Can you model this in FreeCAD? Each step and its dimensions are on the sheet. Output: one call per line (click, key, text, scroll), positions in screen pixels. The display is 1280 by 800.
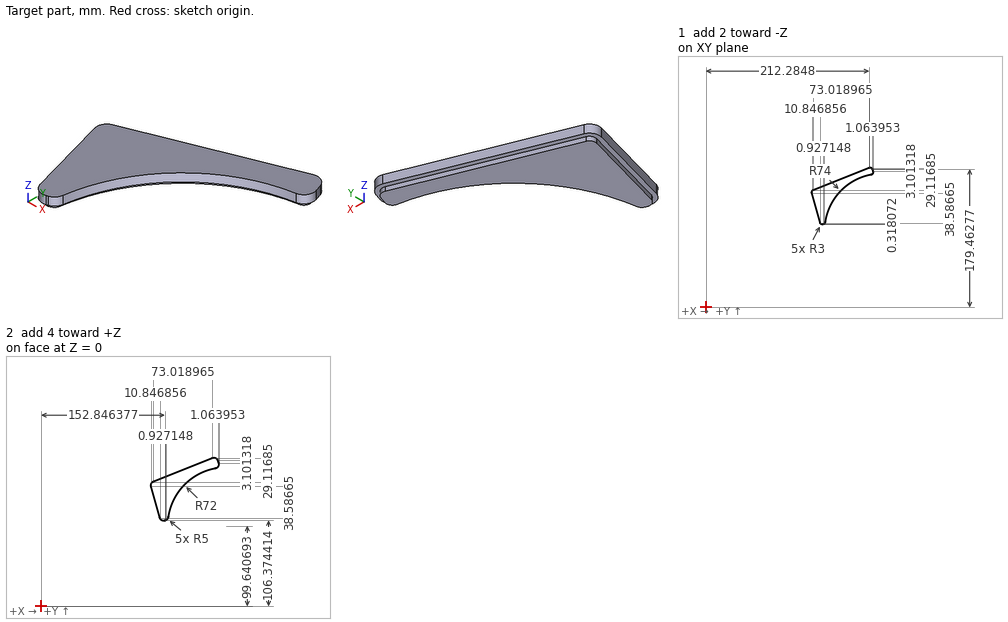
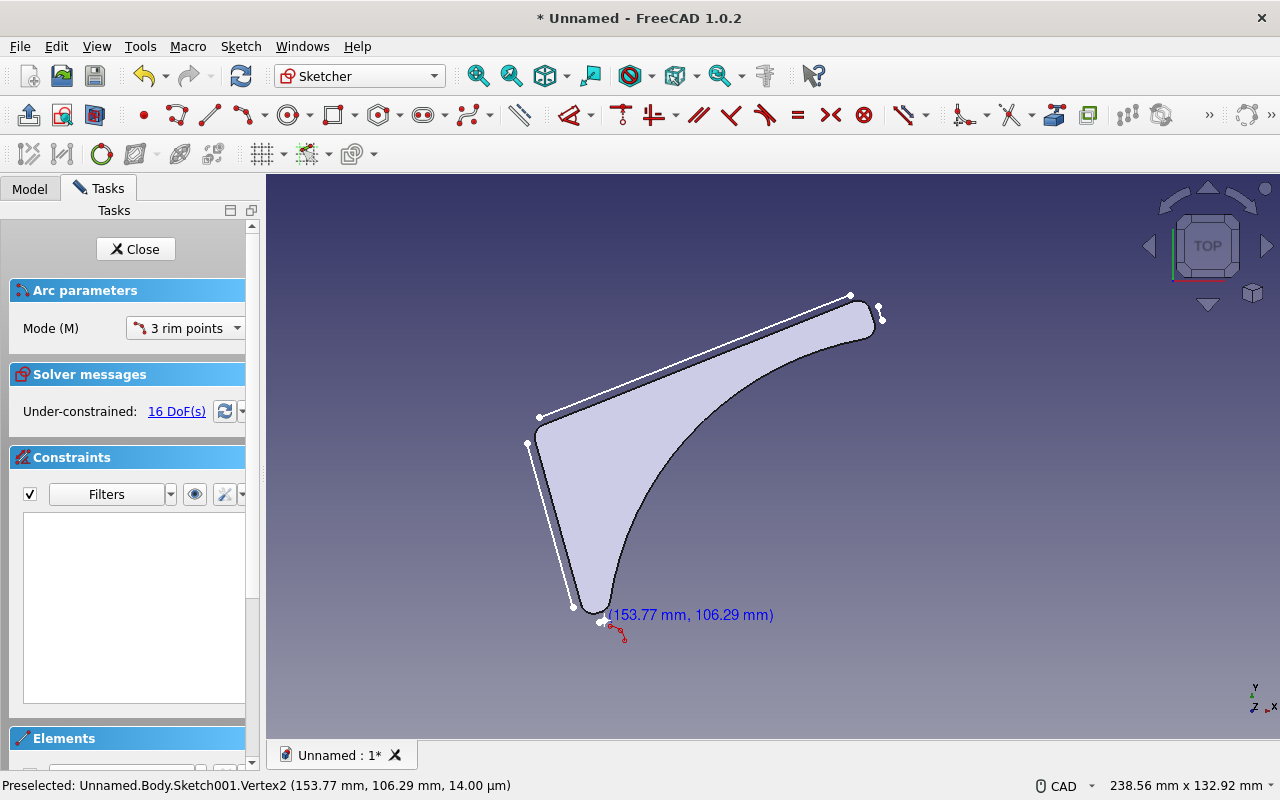
click(618, 603)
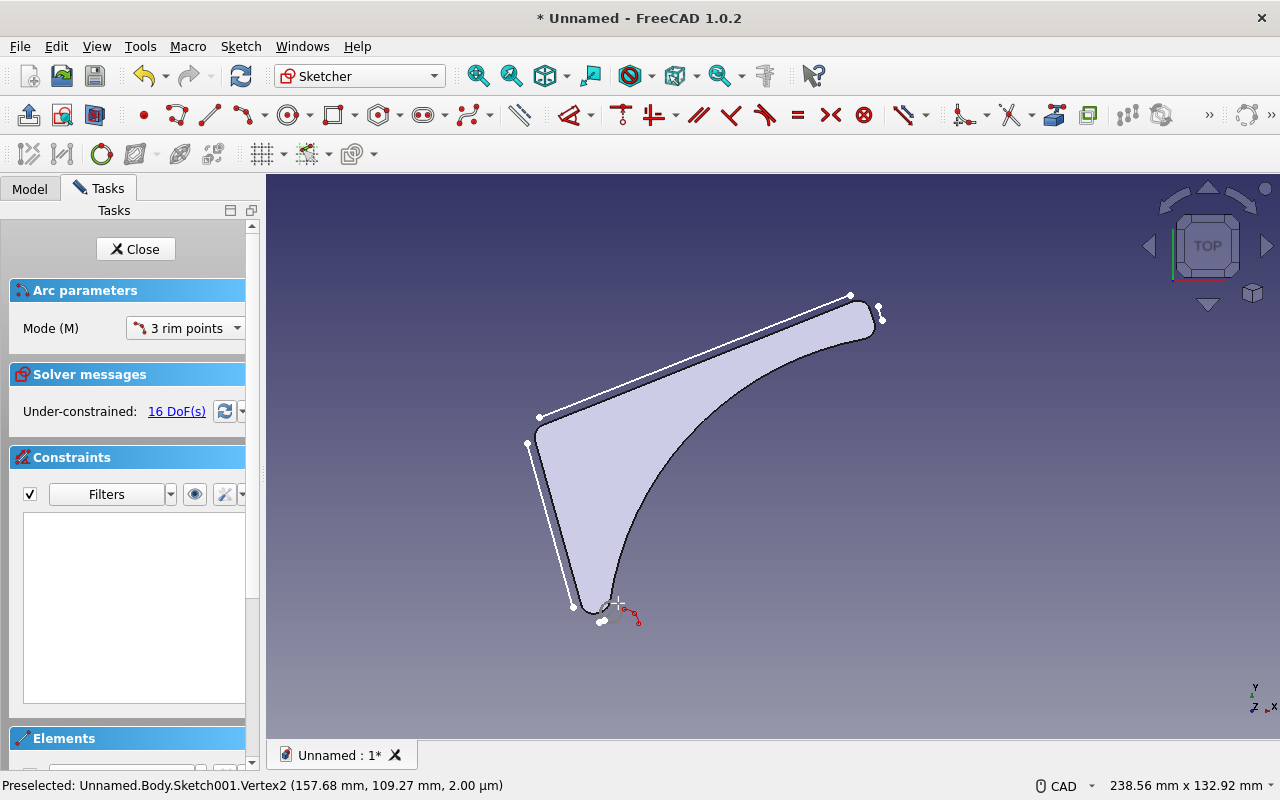
scroll(614, 613, up, 9)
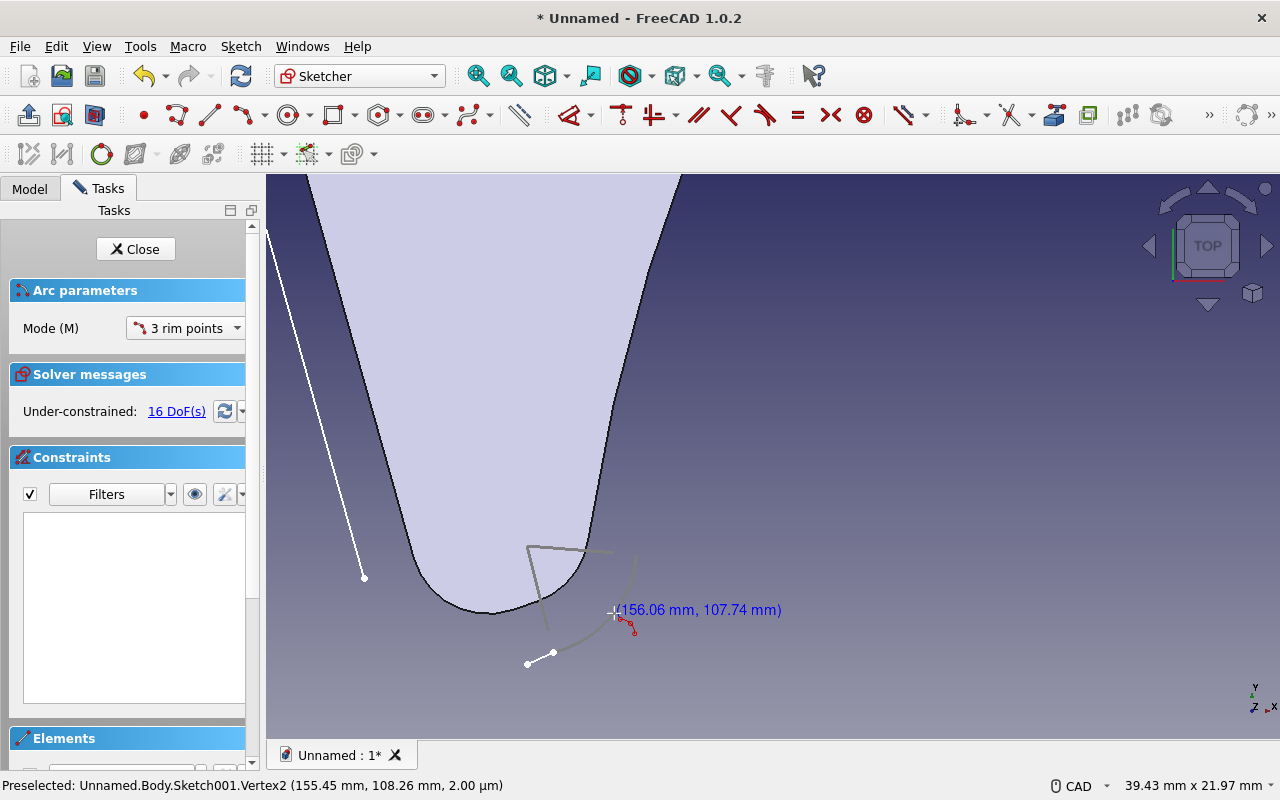
click(611, 611)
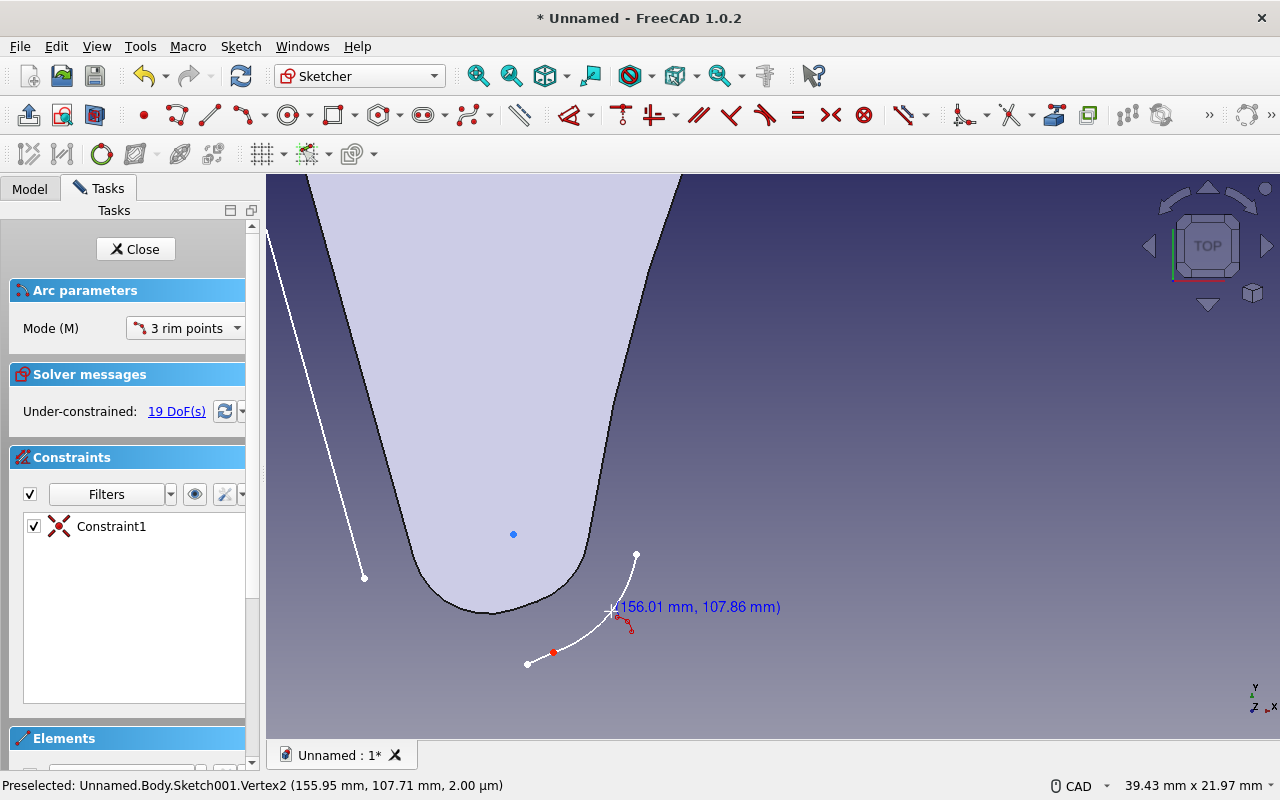
scroll(614, 613, down, 9)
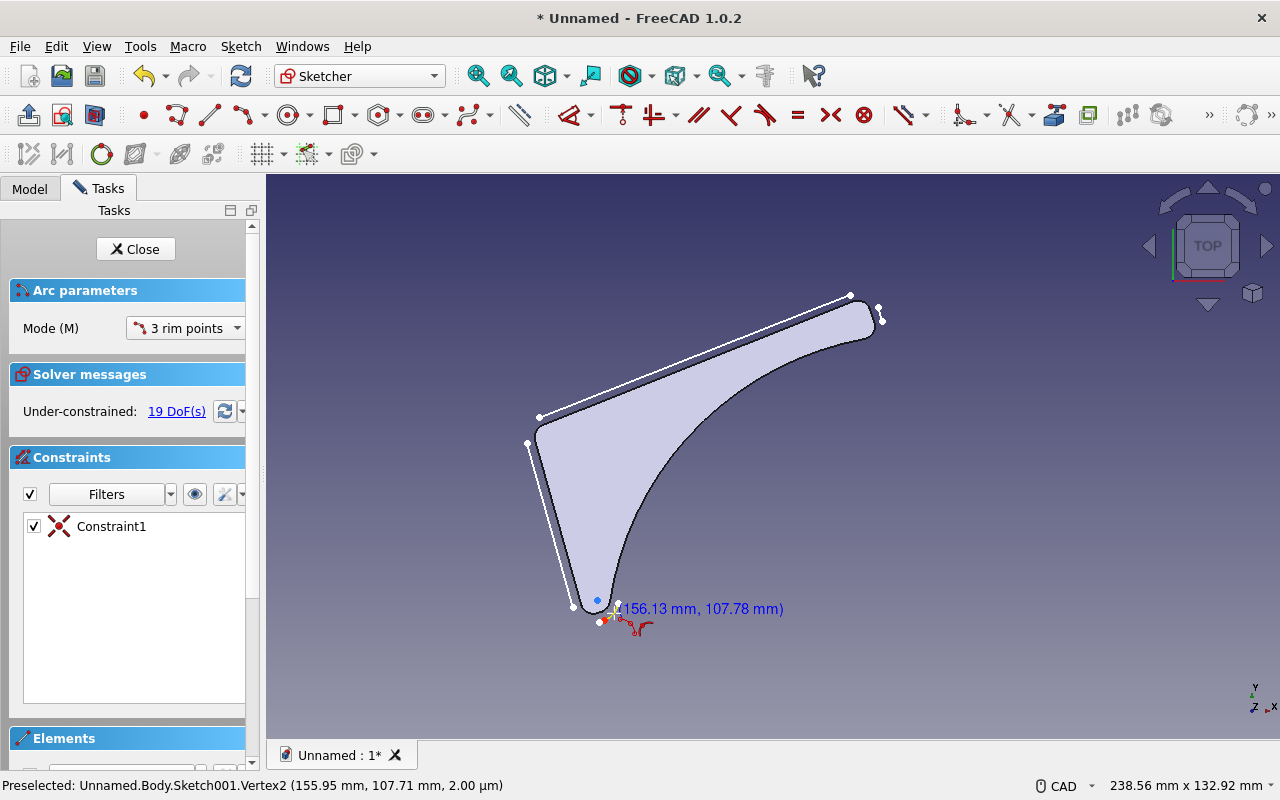
click(618, 604)
click(866, 347)
click(701, 435)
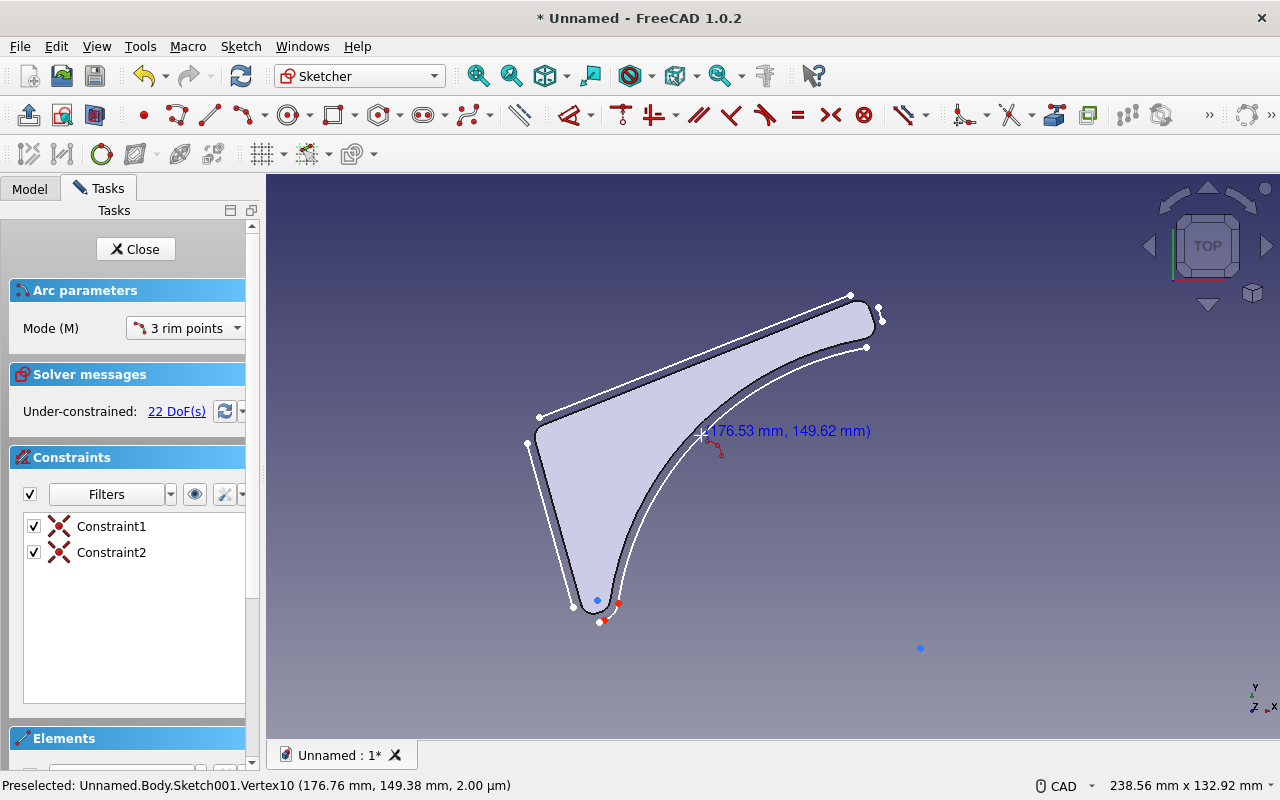
click(866, 348)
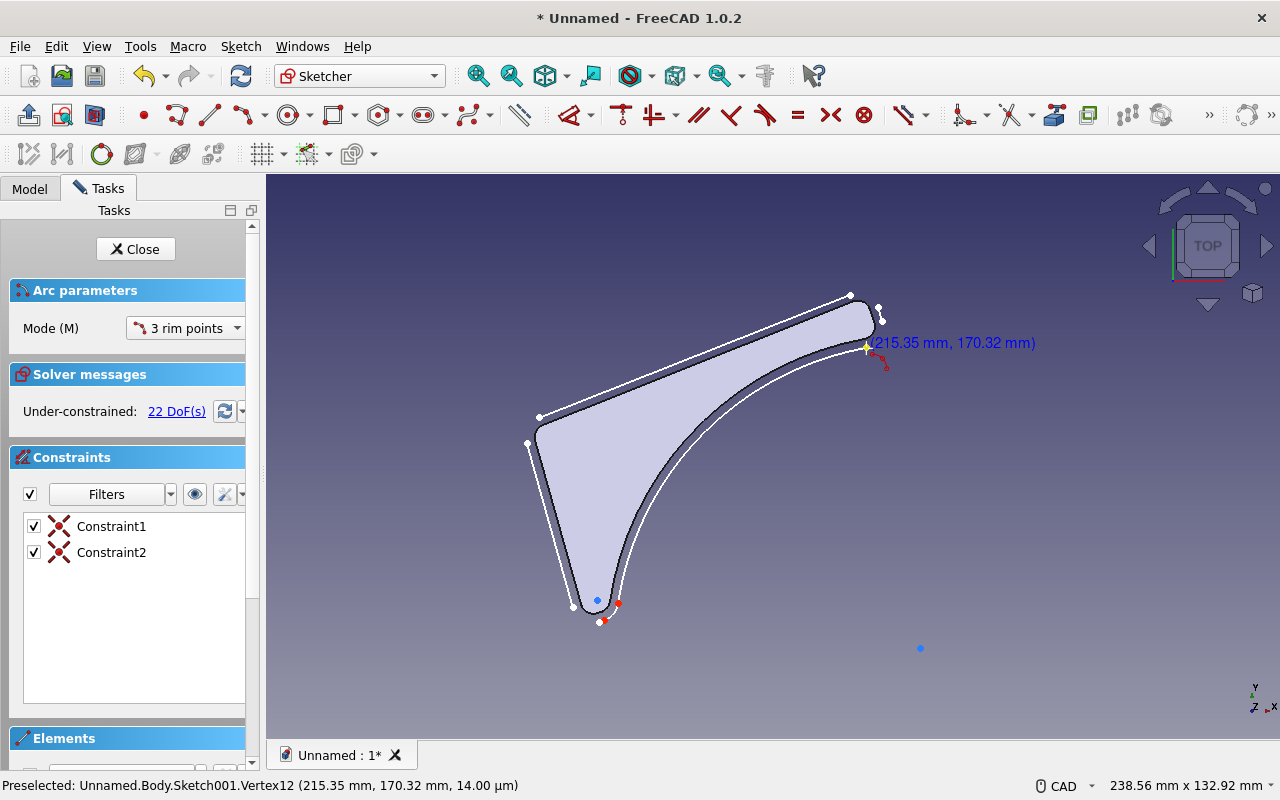
scroll(882, 320, up, 5)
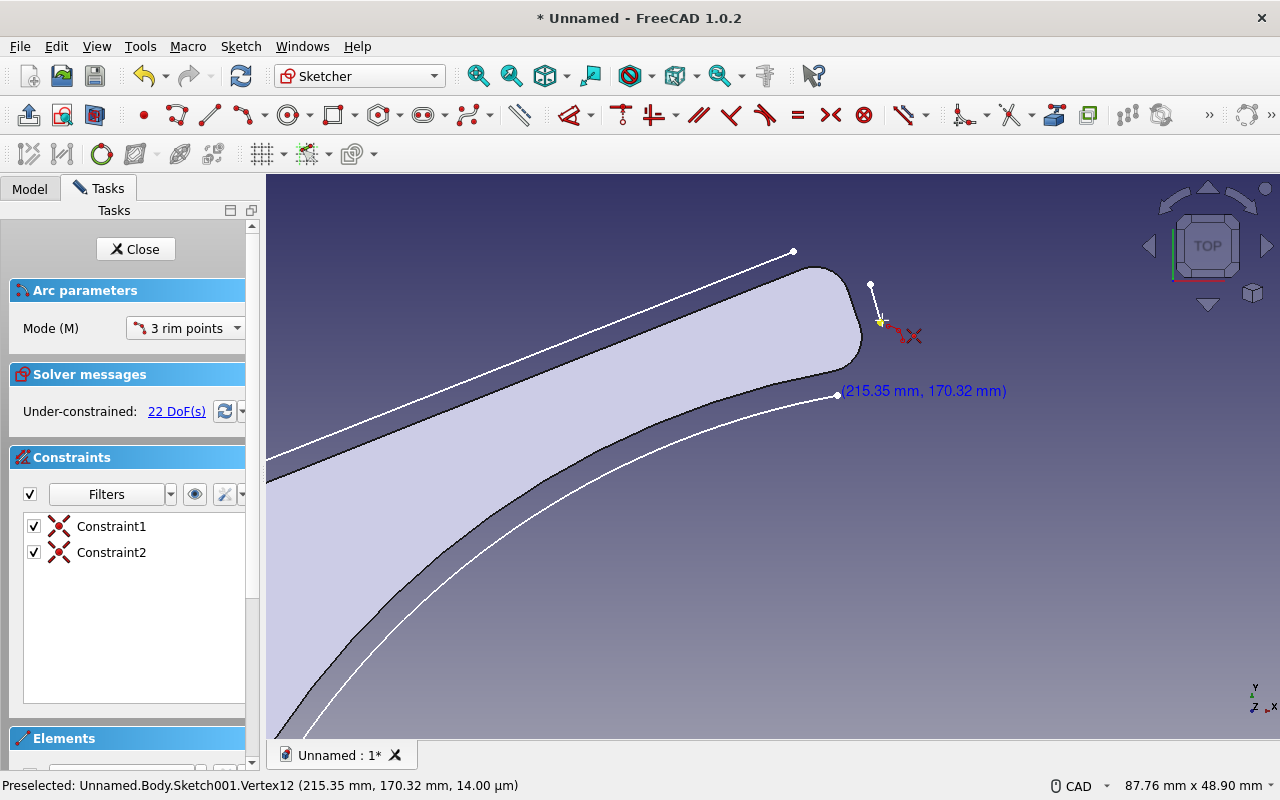
click(881, 322)
click(877, 366)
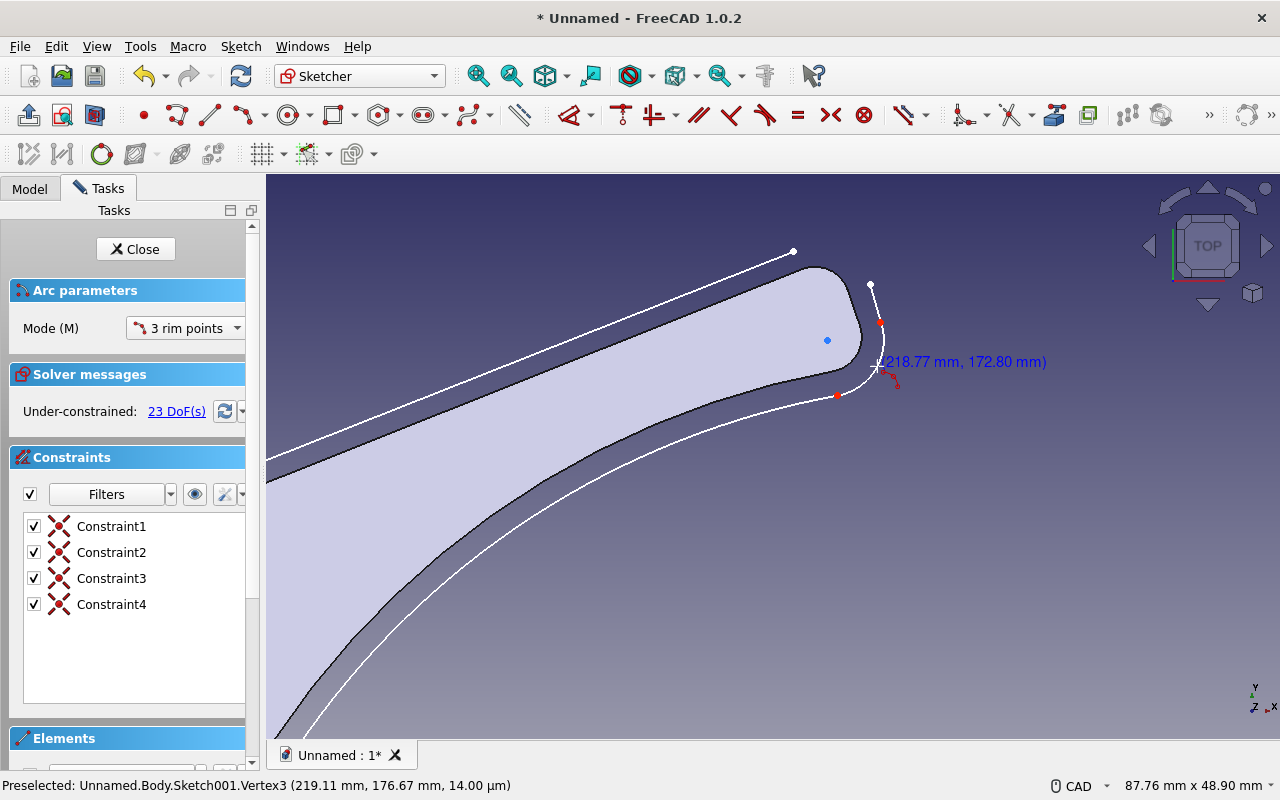
click(870, 284)
click(794, 252)
click(839, 249)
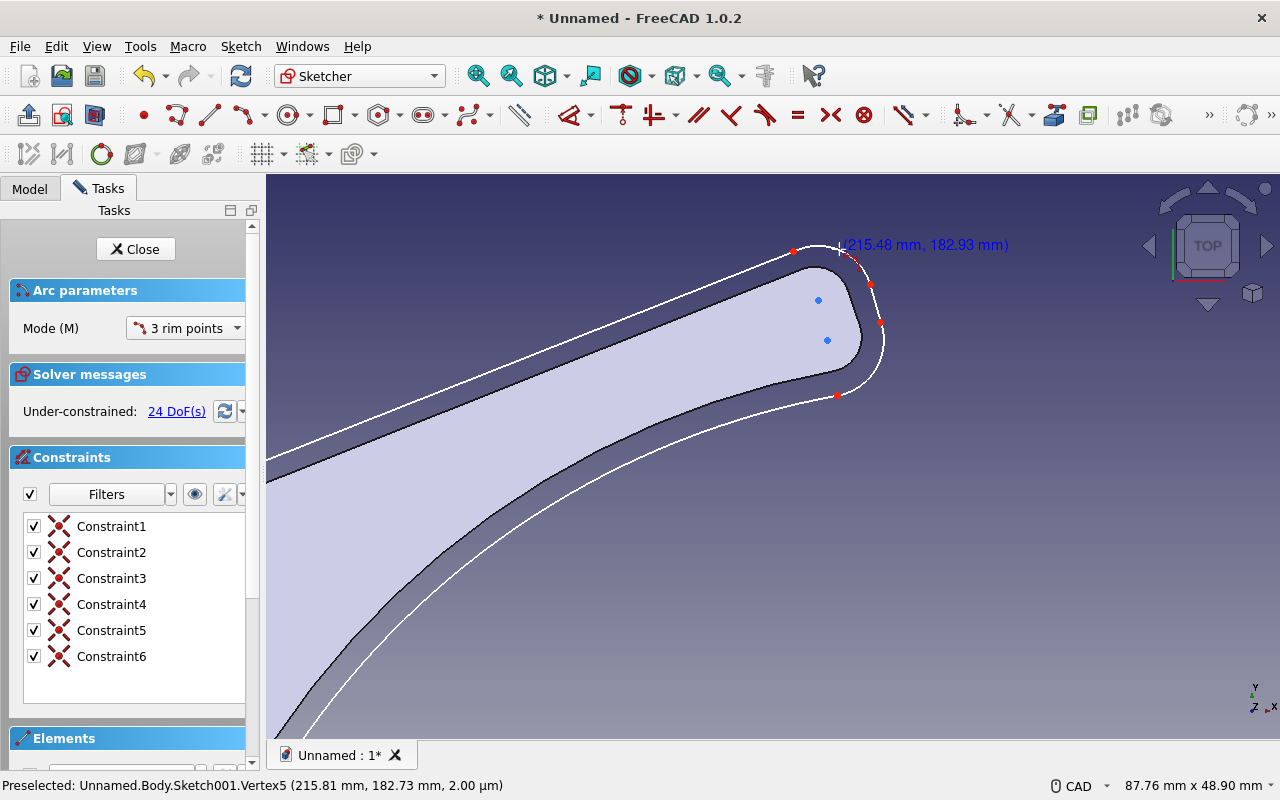
scroll(882, 319, down, 5)